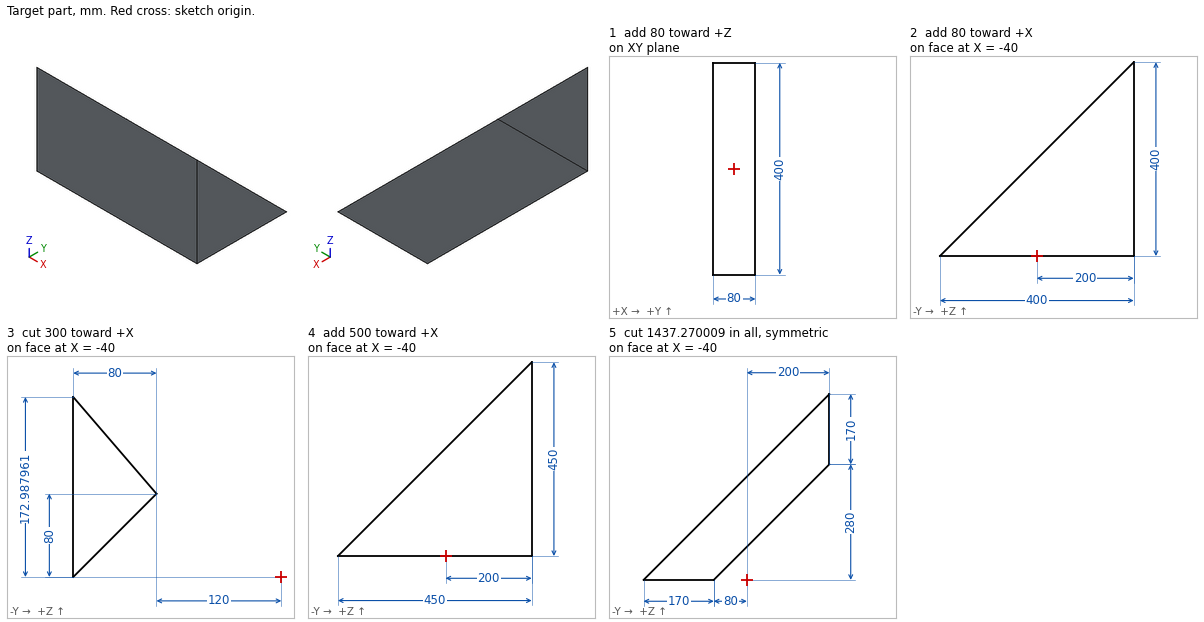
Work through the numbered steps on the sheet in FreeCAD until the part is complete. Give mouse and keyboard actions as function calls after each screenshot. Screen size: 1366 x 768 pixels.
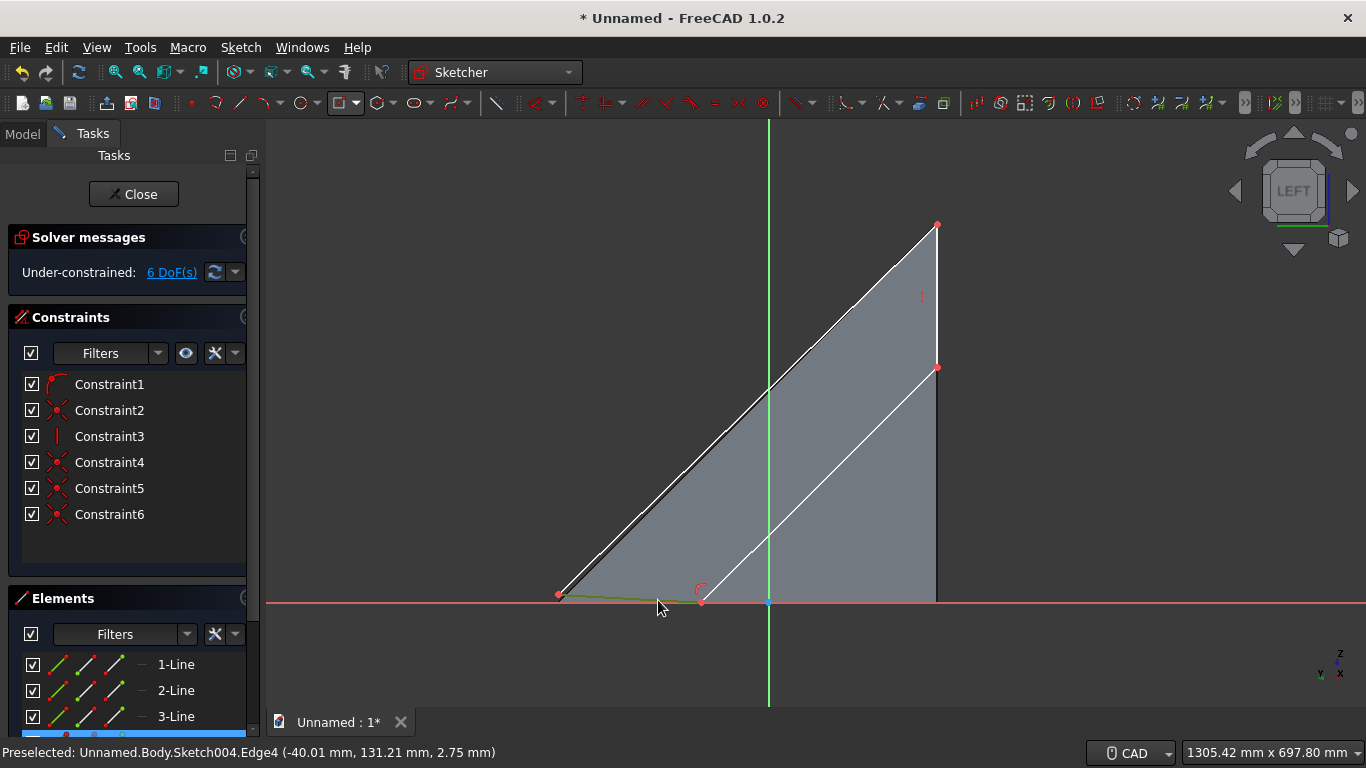
click(624, 104)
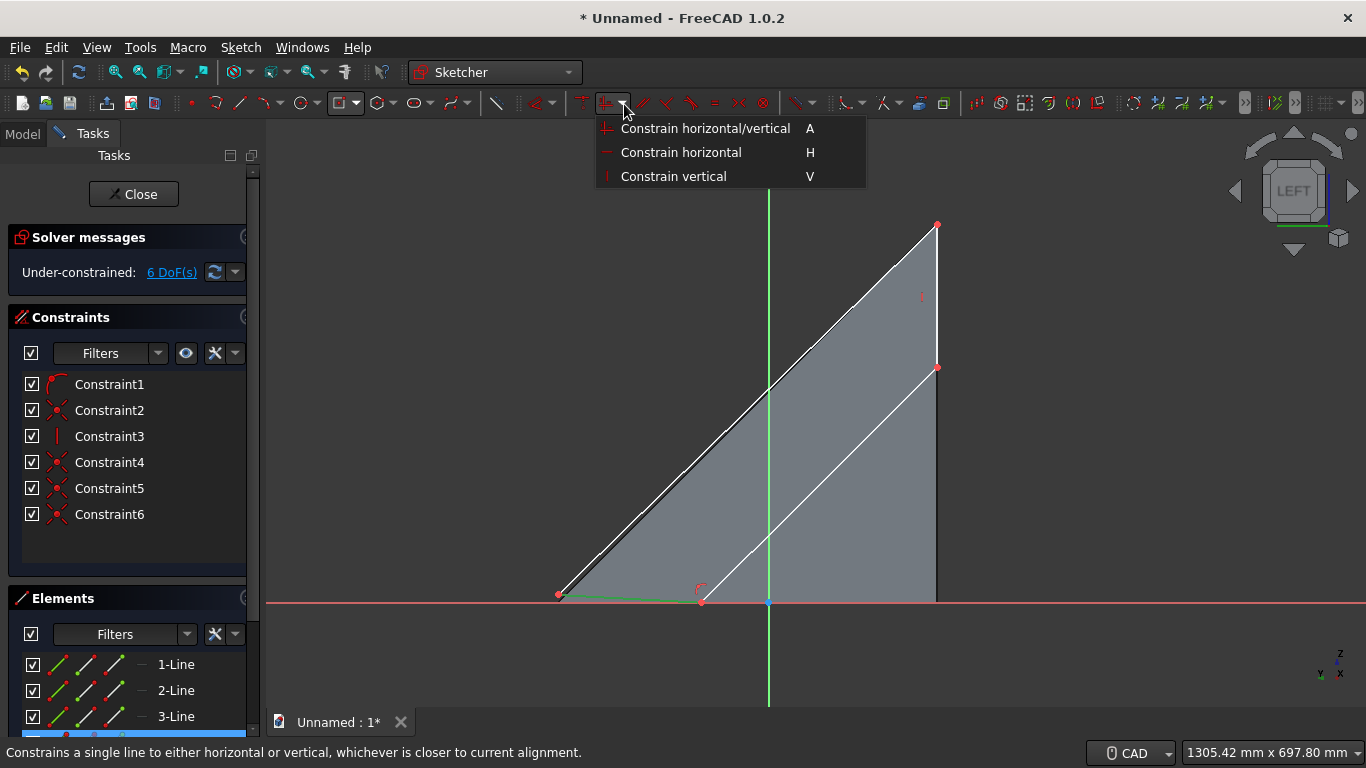
click(731, 152)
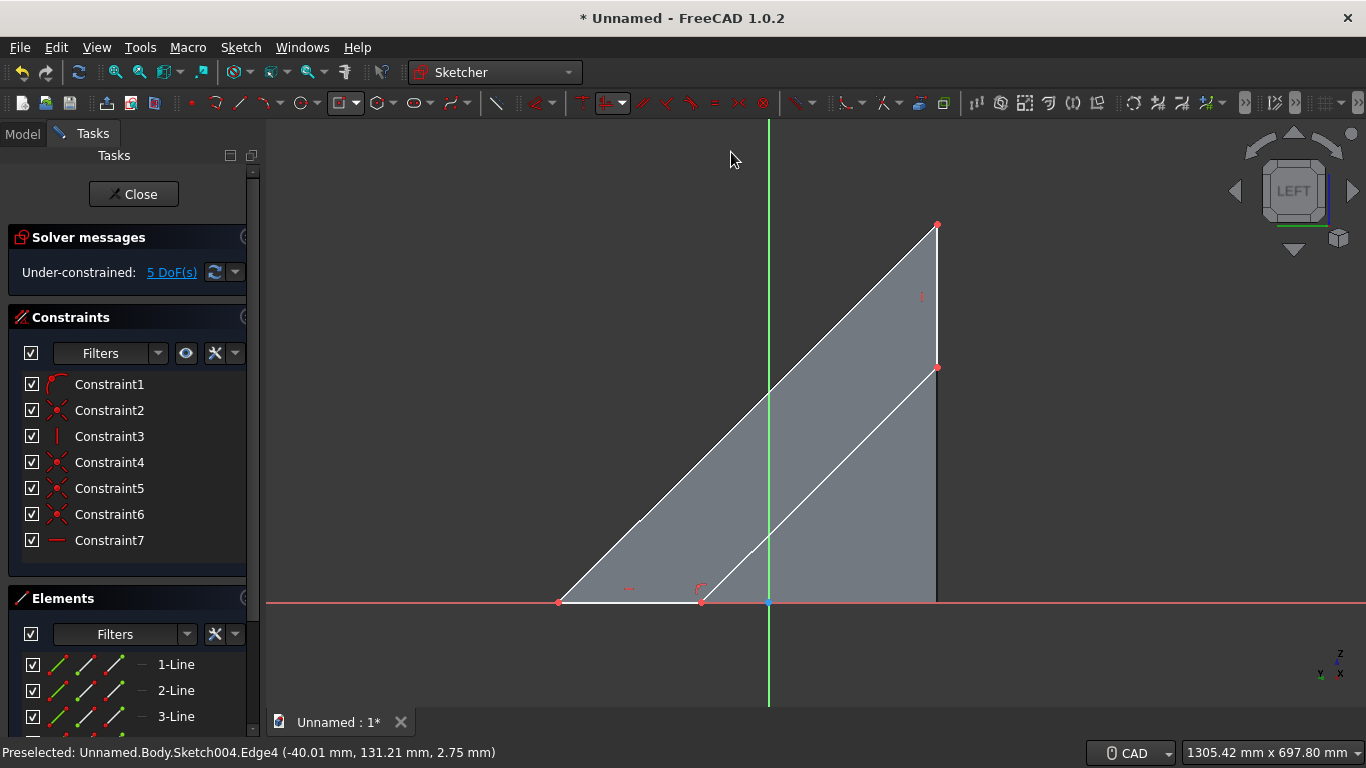
click(536, 104)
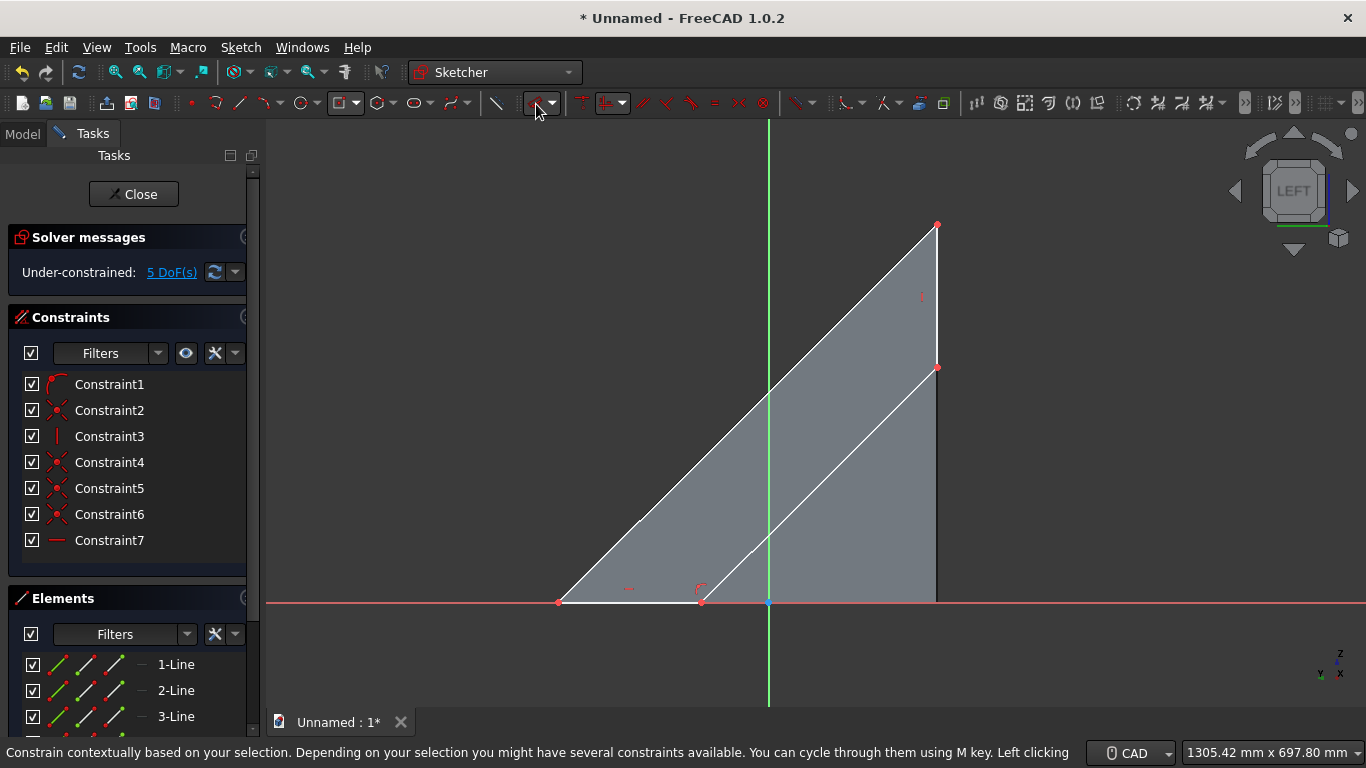
click(937, 325)
click(971, 296)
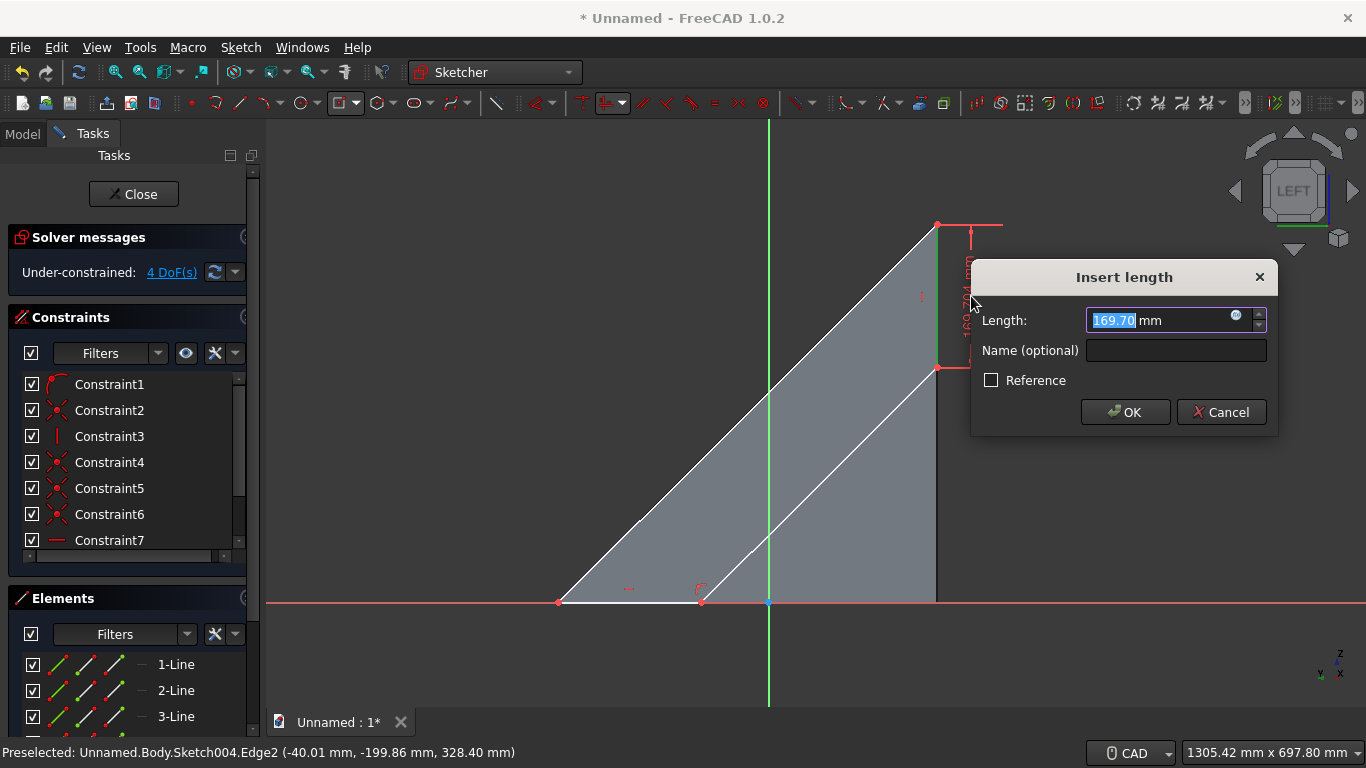
text(170)
key(Return)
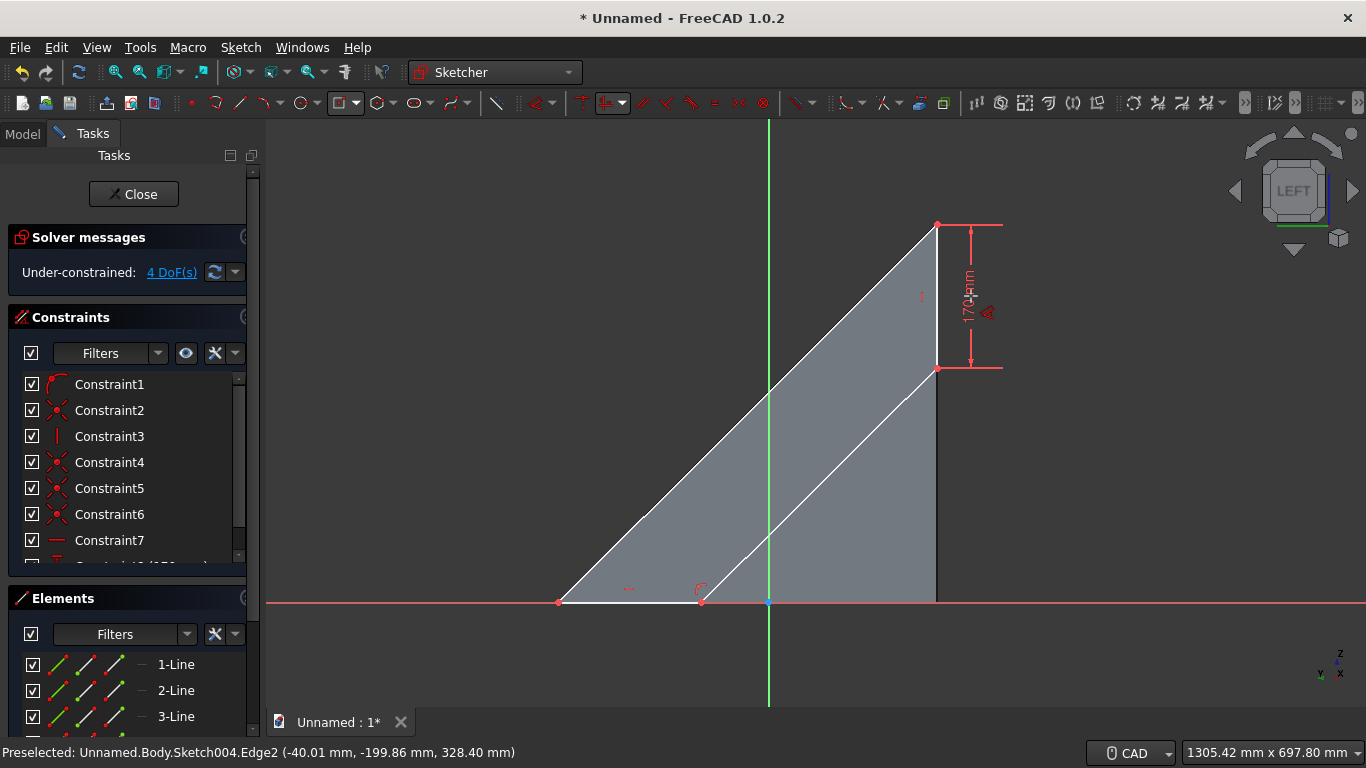
click(601, 603)
click(629, 637)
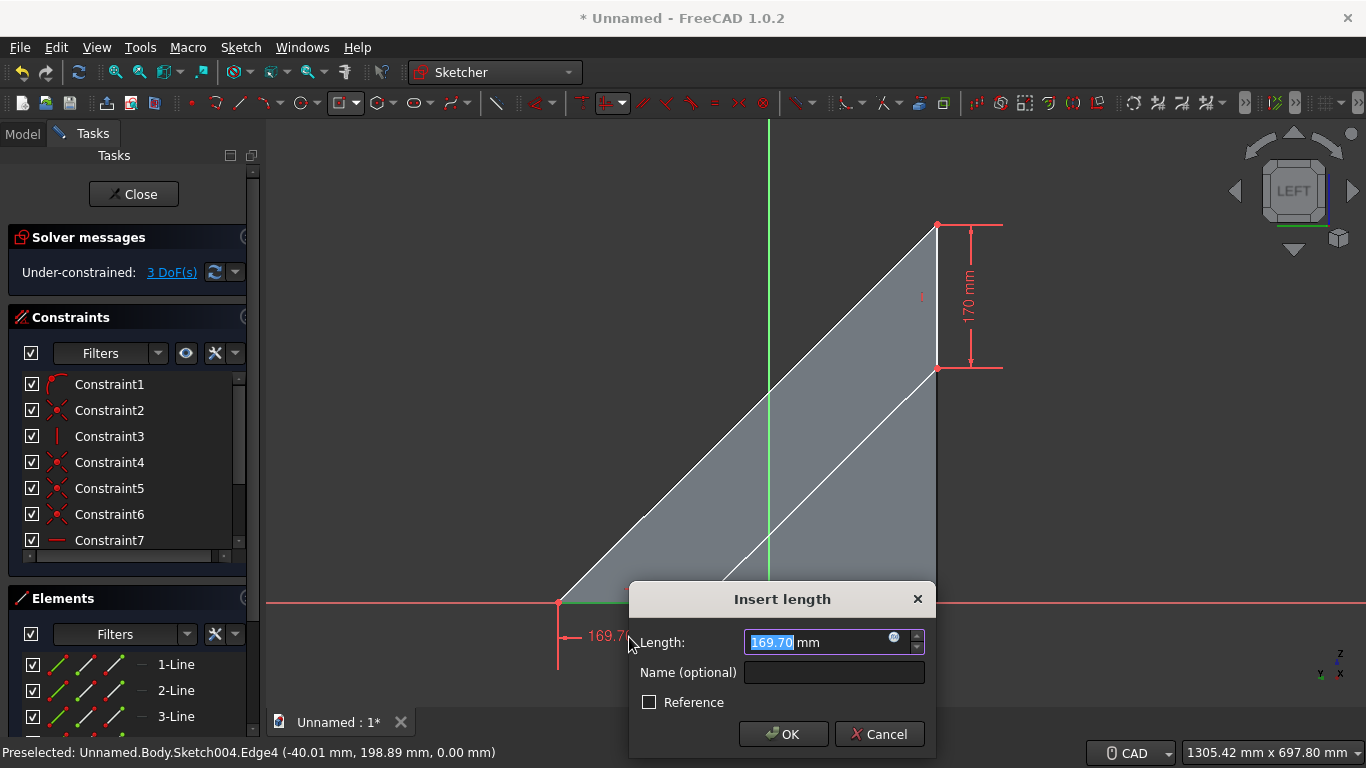
text(170)
key(Return)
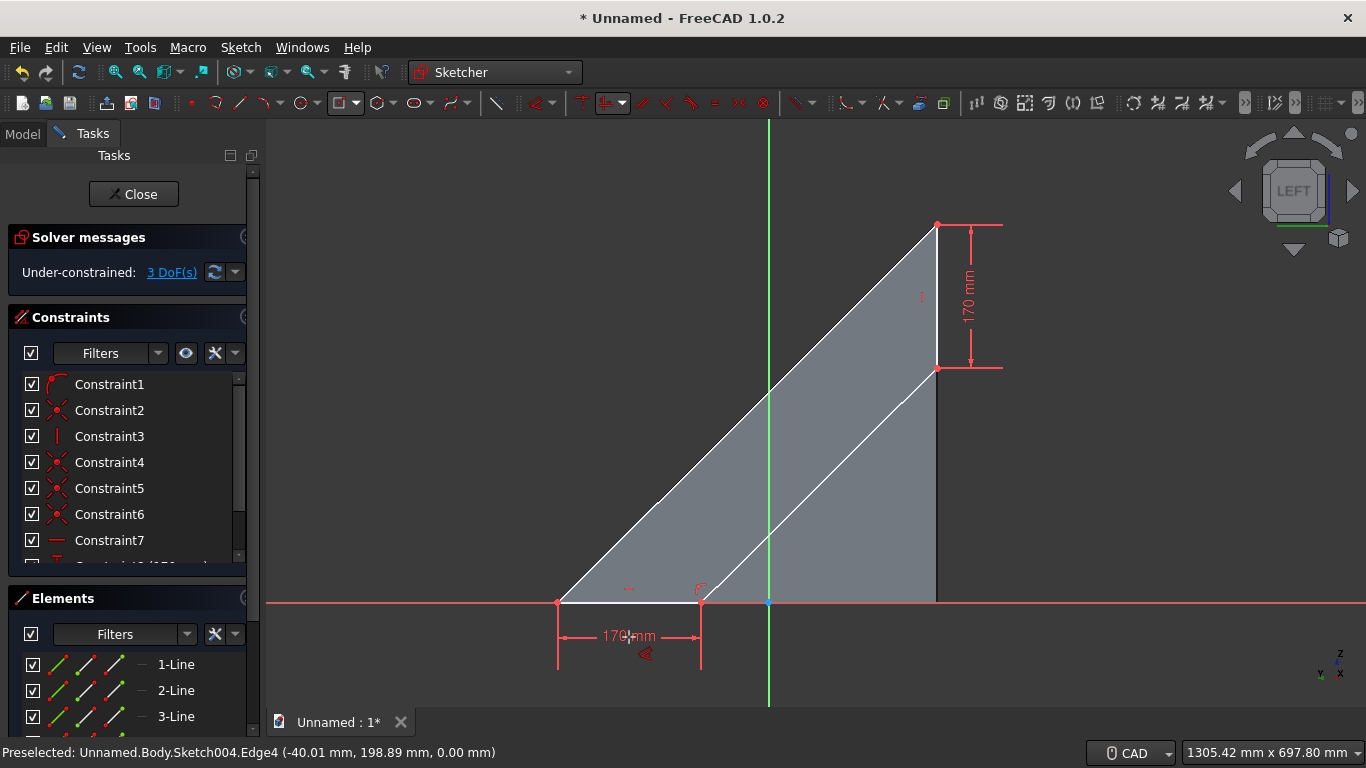
click(701, 603)
click(735, 637)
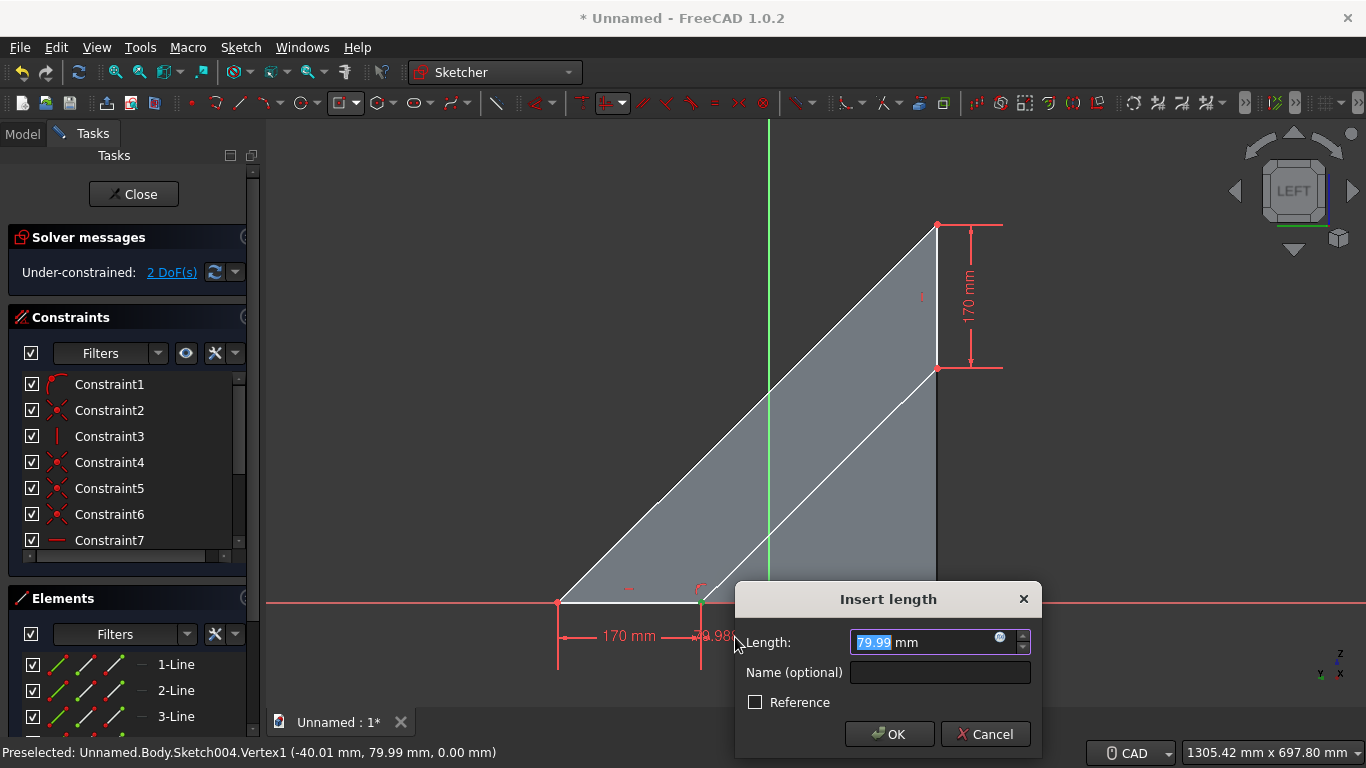
text(80)
key(Return)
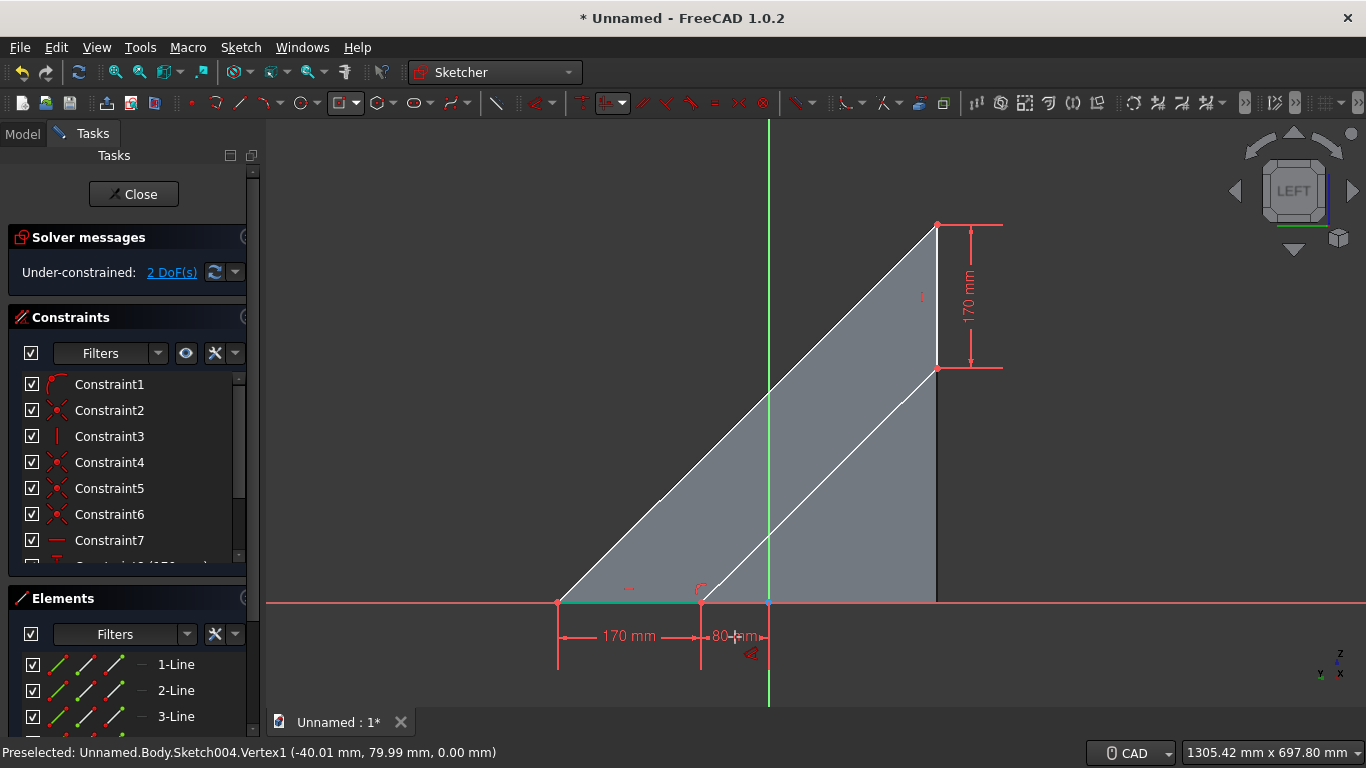
click(937, 368)
click(853, 637)